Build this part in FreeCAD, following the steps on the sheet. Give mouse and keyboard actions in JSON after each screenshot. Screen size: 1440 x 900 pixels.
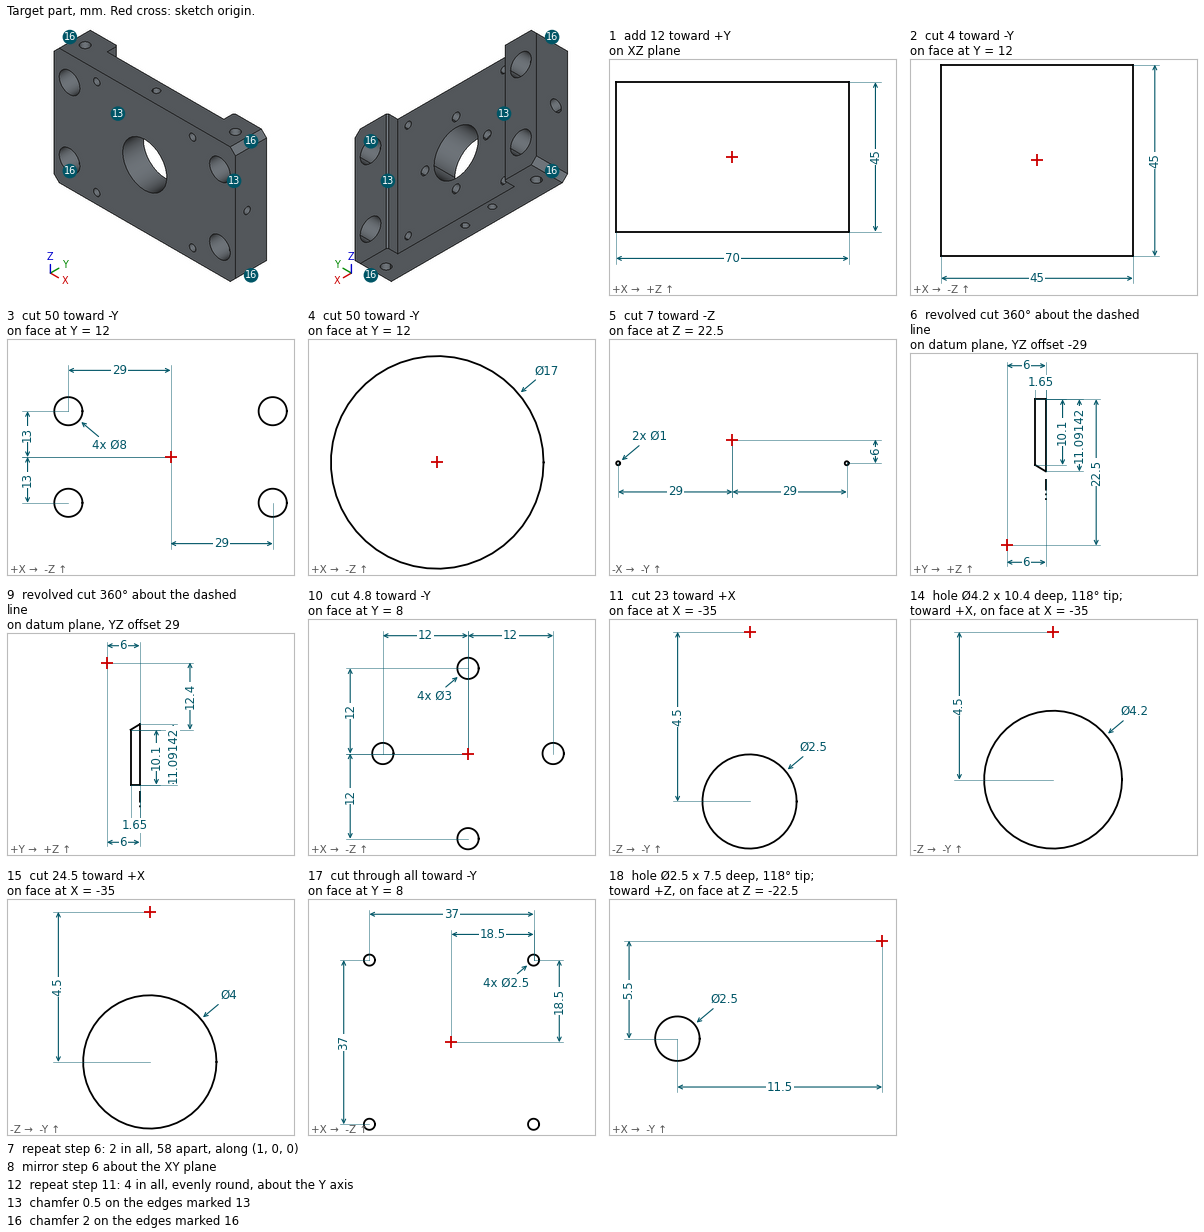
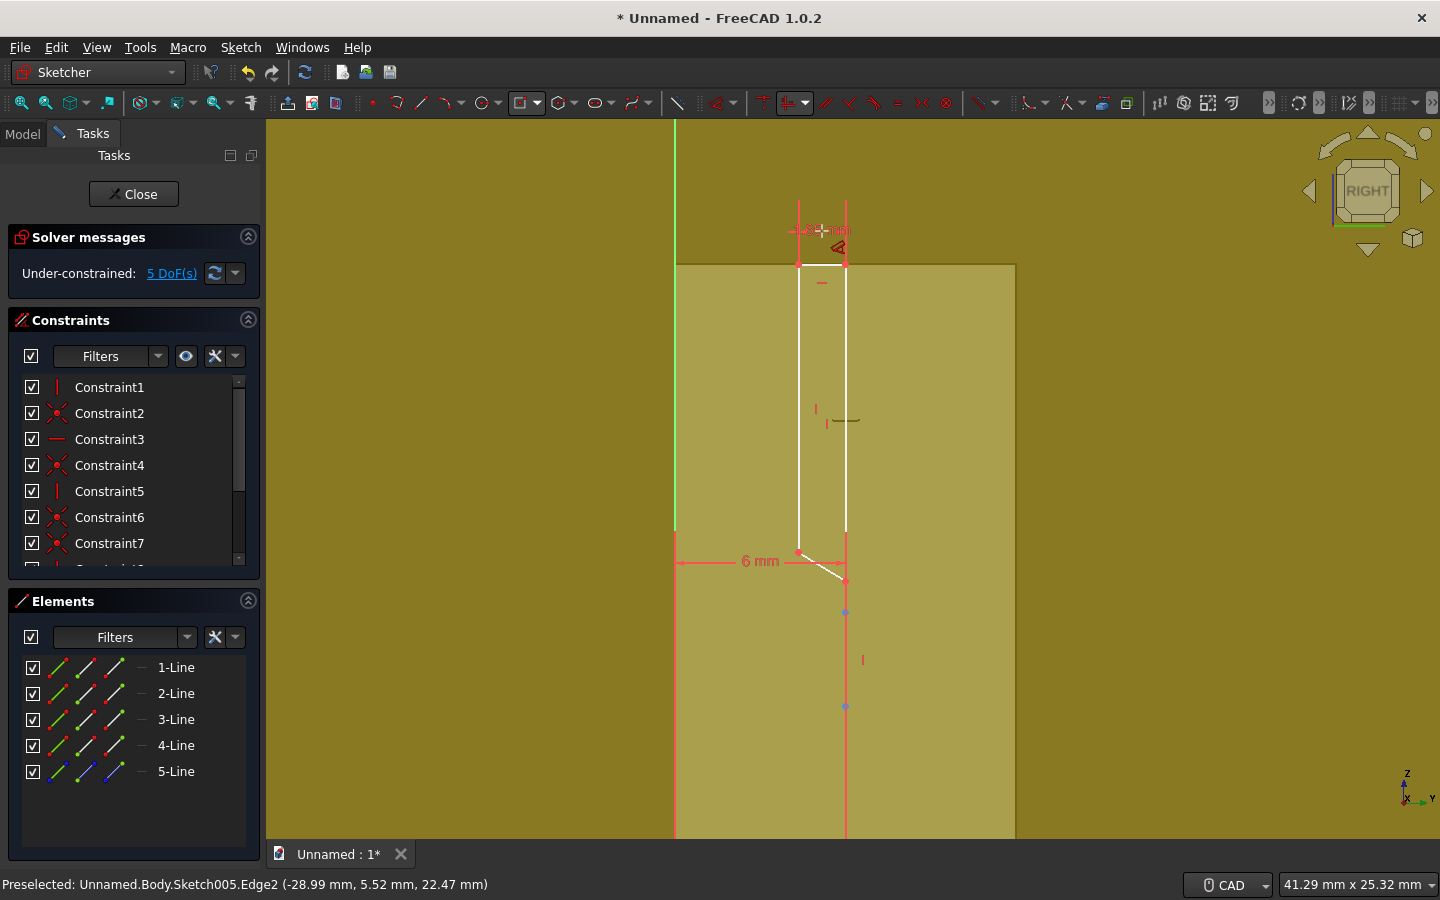
{"action": "left_click", "coordinate": [799, 351]}
{"action": "left_click", "coordinate": [765, 409]}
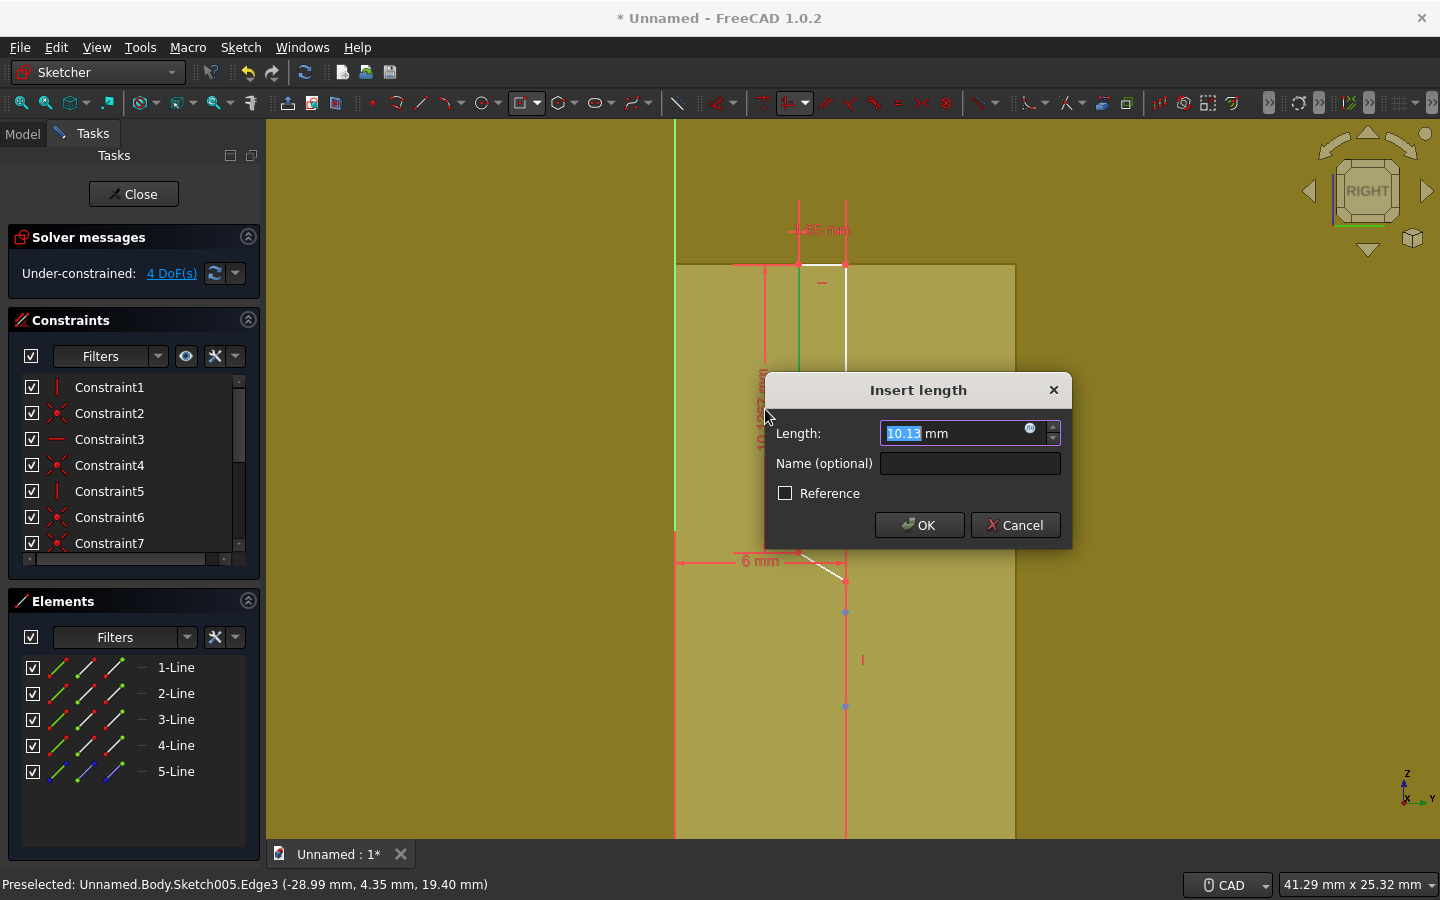
{"action": "type", "text": "10.1"}
{"action": "key", "text": "Return"}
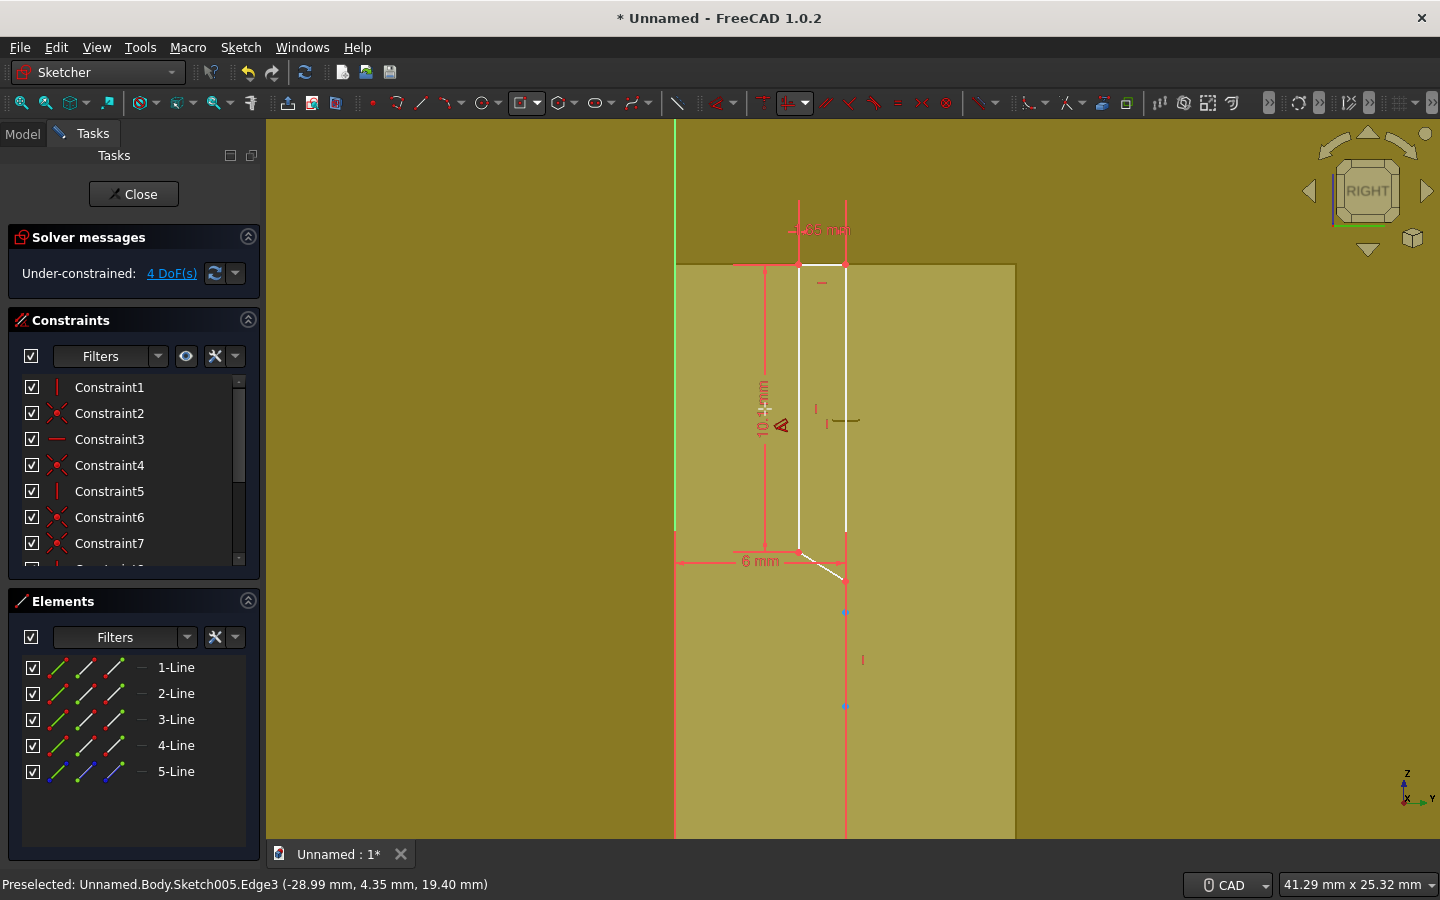
{"action": "left_click", "coordinate": [846, 265]}
{"action": "left_click", "coordinate": [880, 538]}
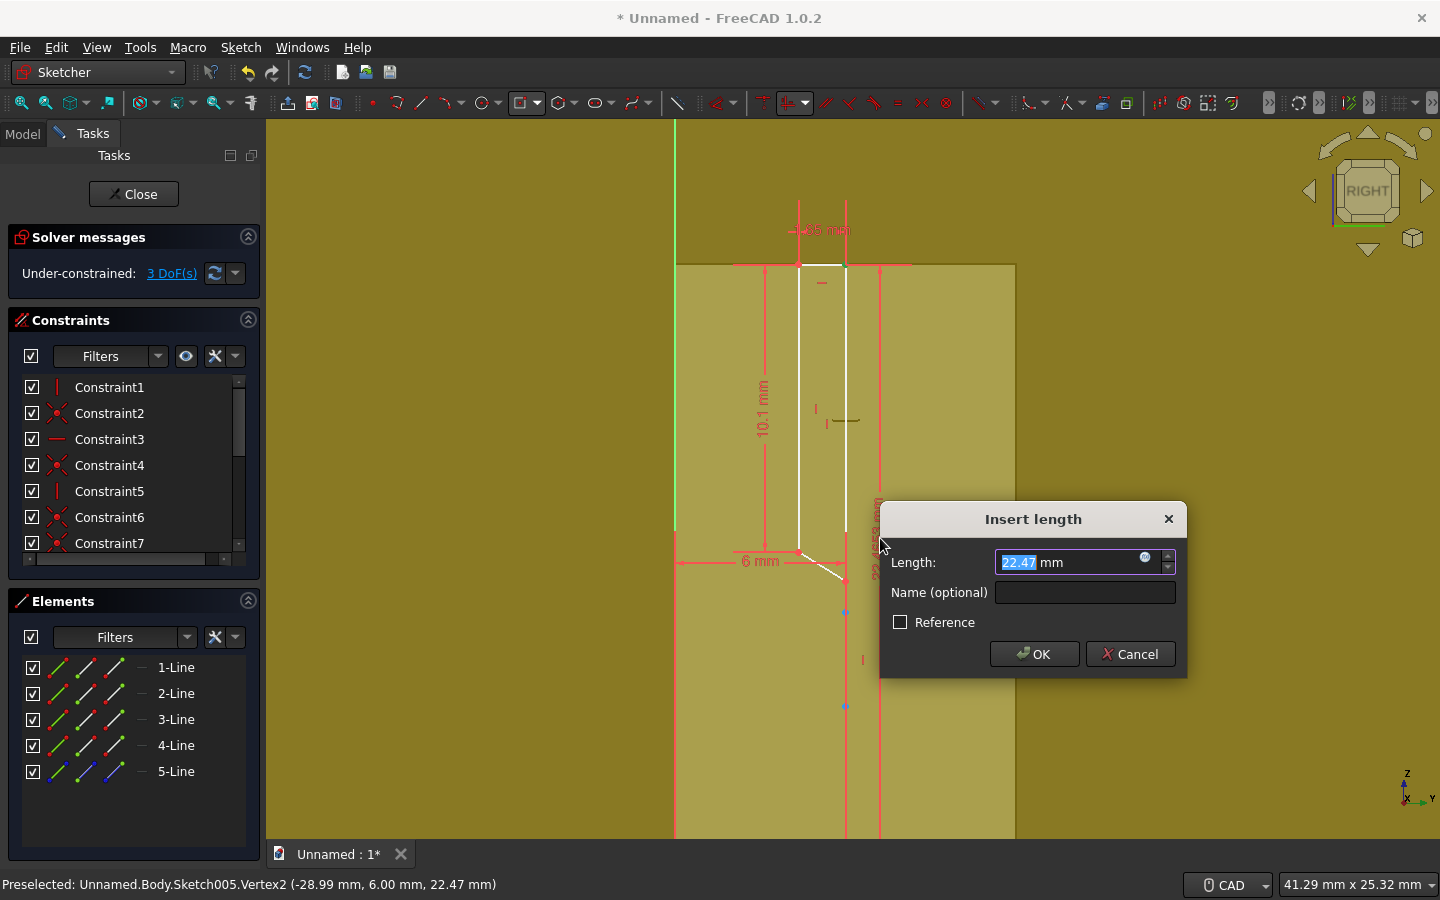
{"action": "type", "text": "22.5"}
{"action": "key", "text": "Return"}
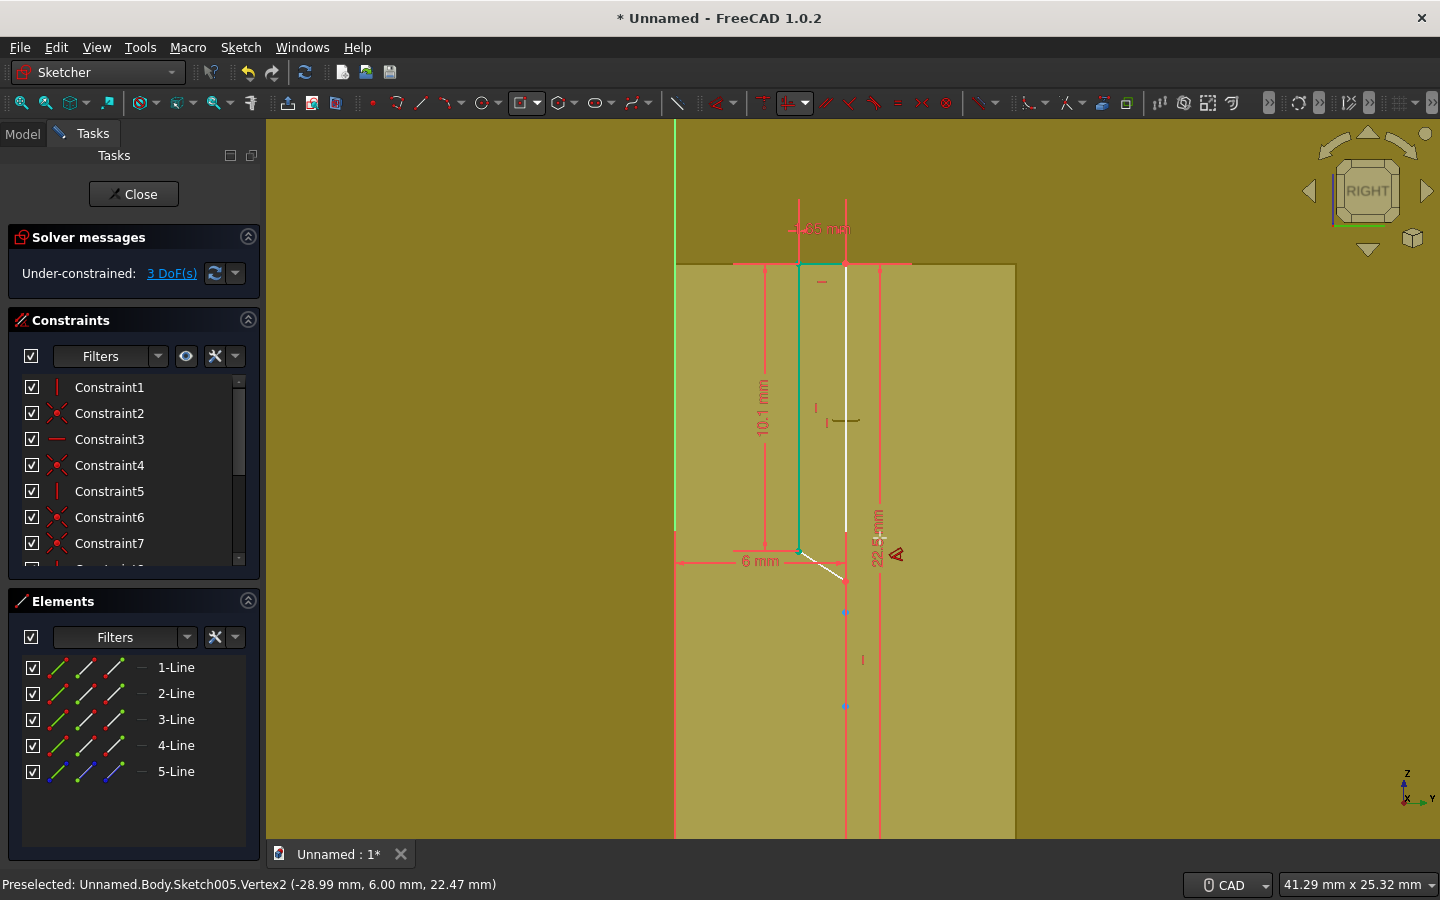
{"action": "left_click", "coordinate": [846, 486]}
{"action": "left_click", "coordinate": [880, 423]}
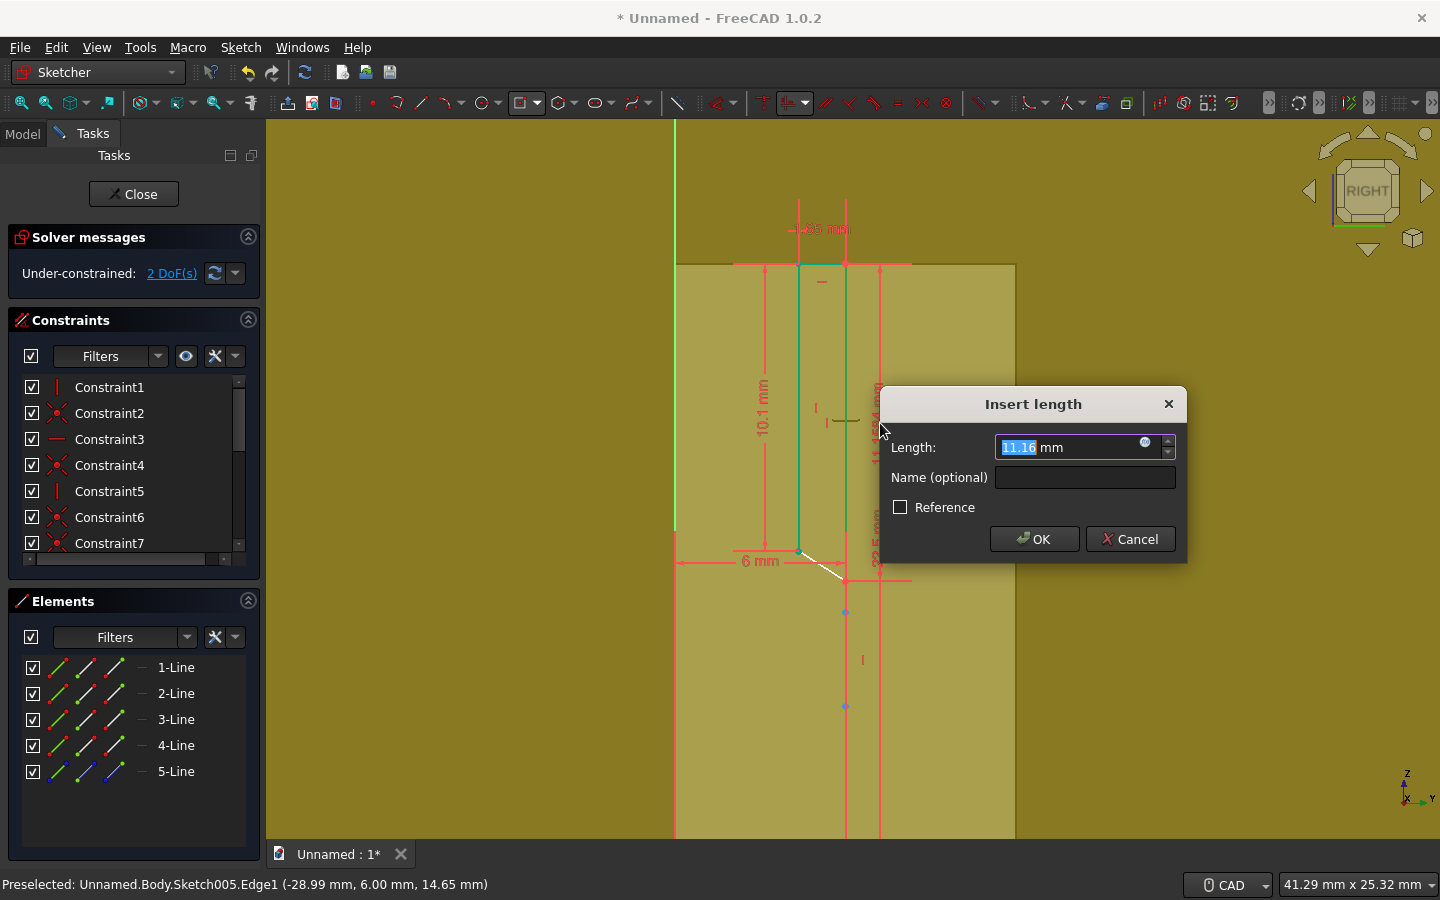
{"action": "type", "text": "11.09142"}
{"action": "key", "text": "Return"}
{"action": "key", "text": "Escape"}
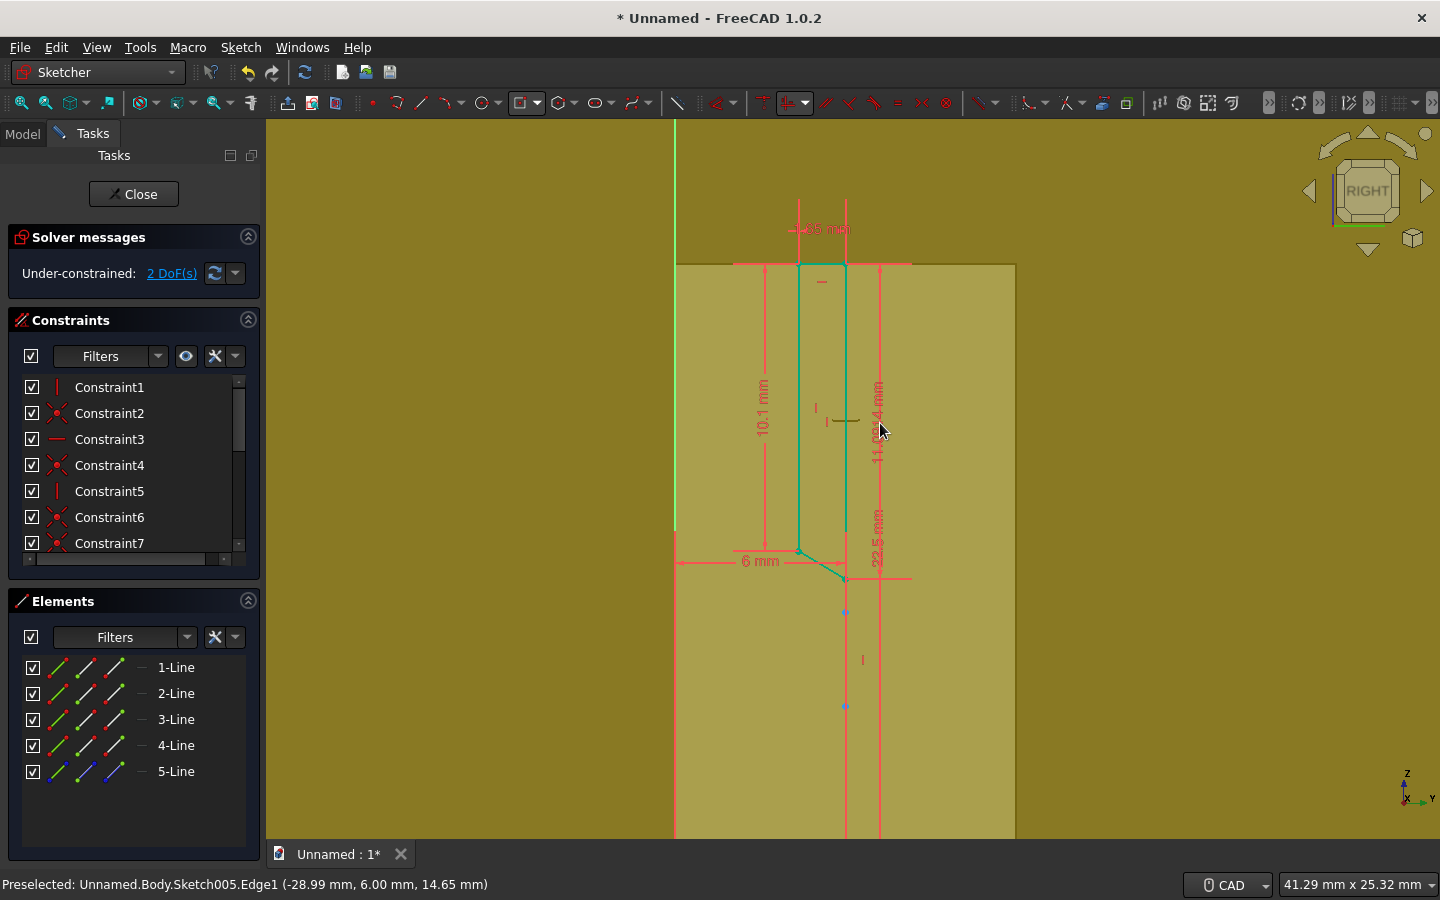
{"action": "left_click", "coordinate": [134, 194]}